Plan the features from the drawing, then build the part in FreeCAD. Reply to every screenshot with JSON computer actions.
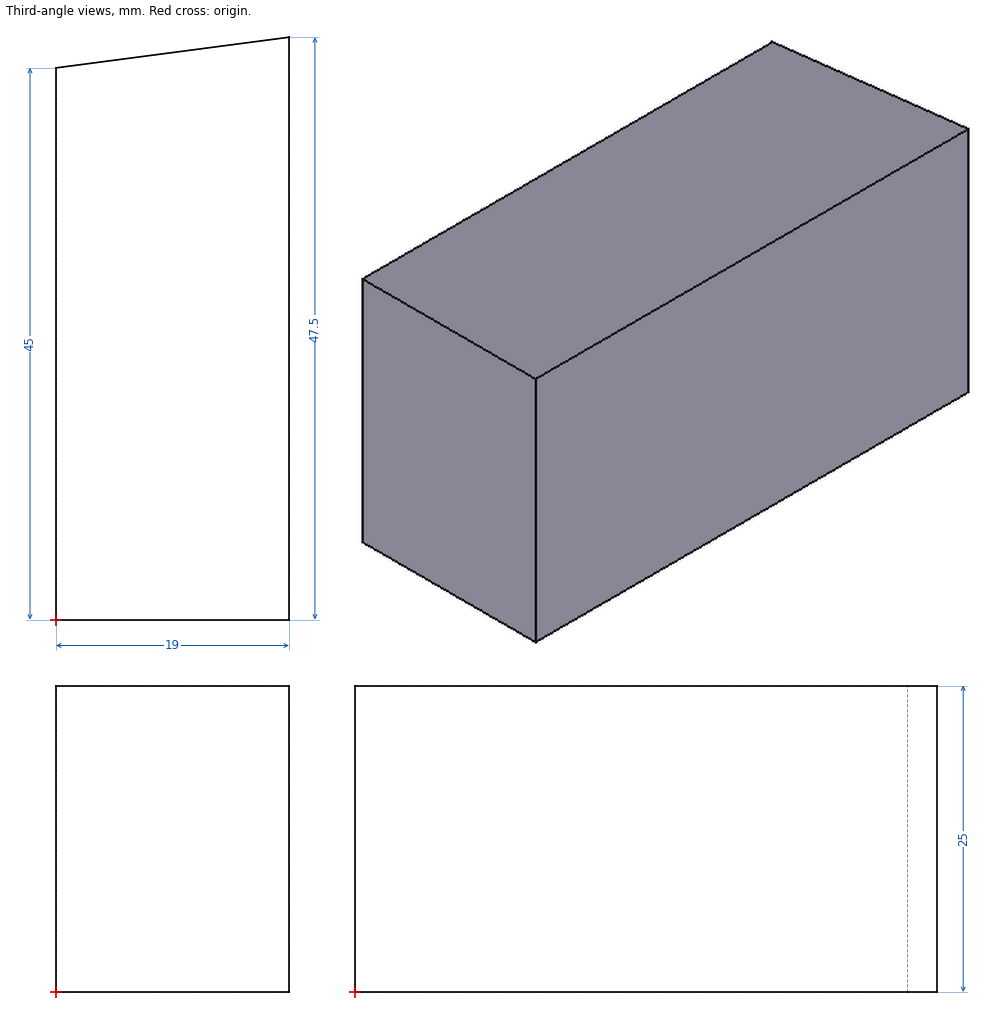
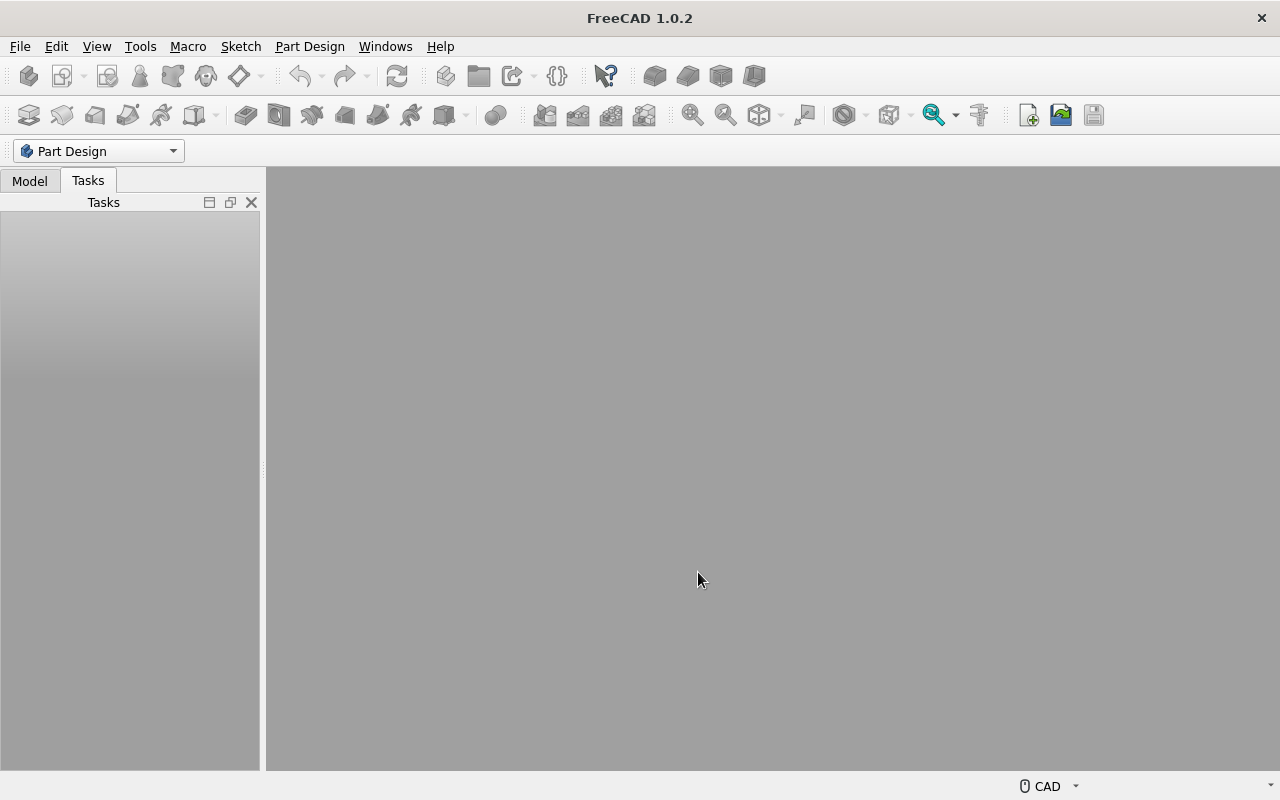
{"action": "key", "text": "ctrl+n"}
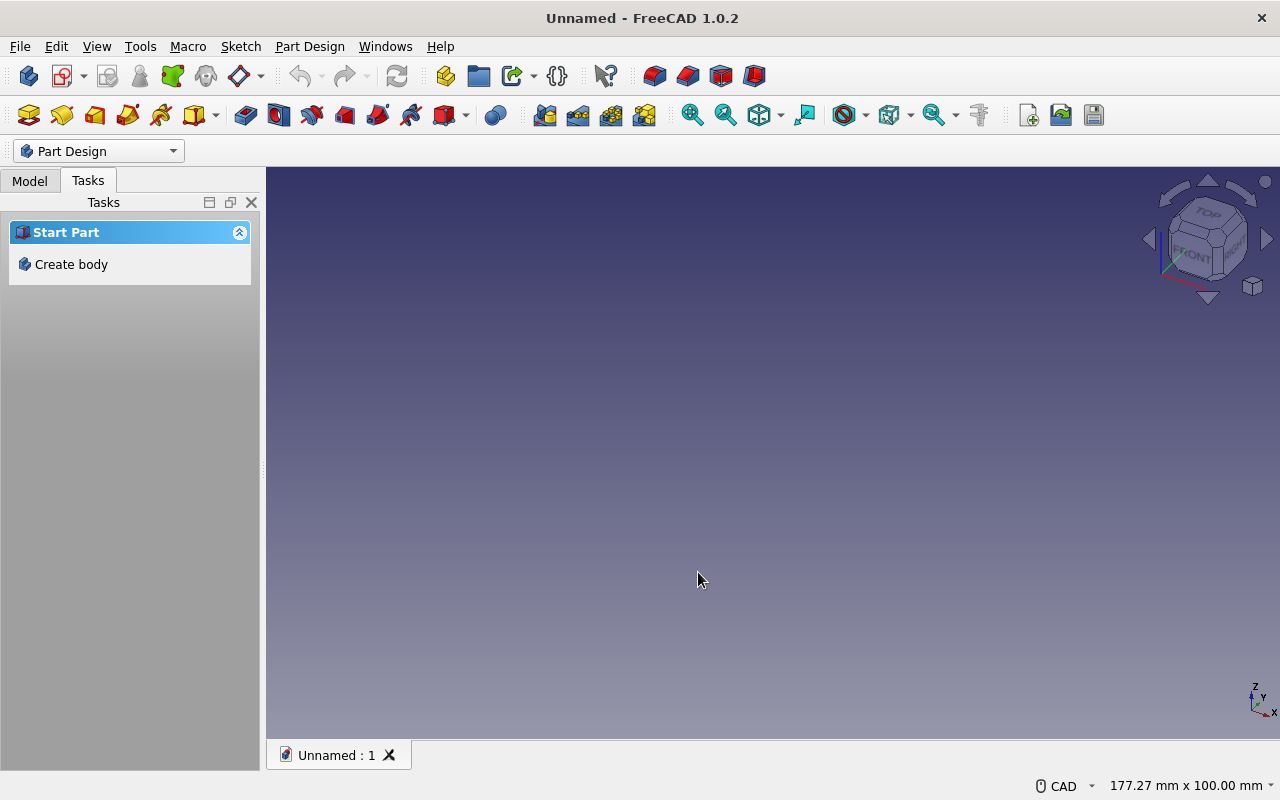
{"action": "left_click", "coordinate": [62, 76]}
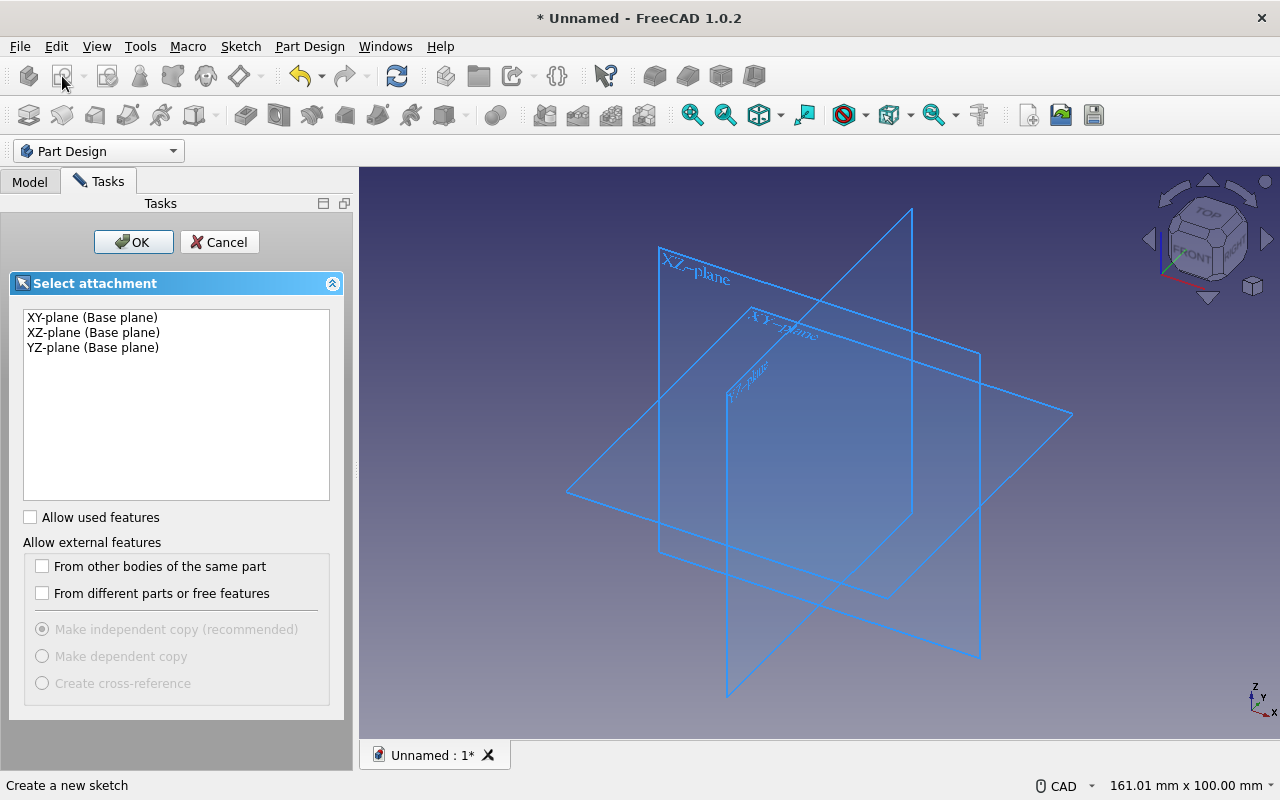
{"action": "left_click", "coordinate": [84, 318]}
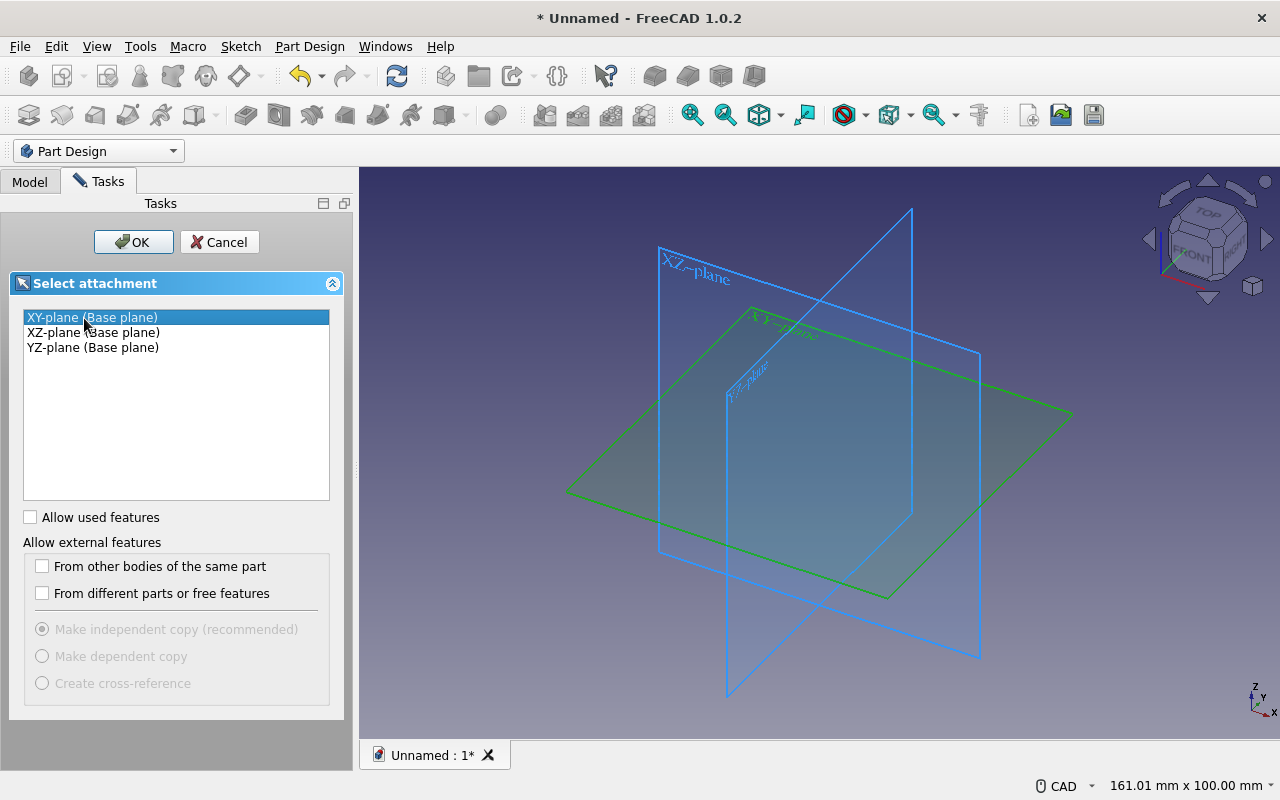
{"action": "left_click", "coordinate": [134, 242]}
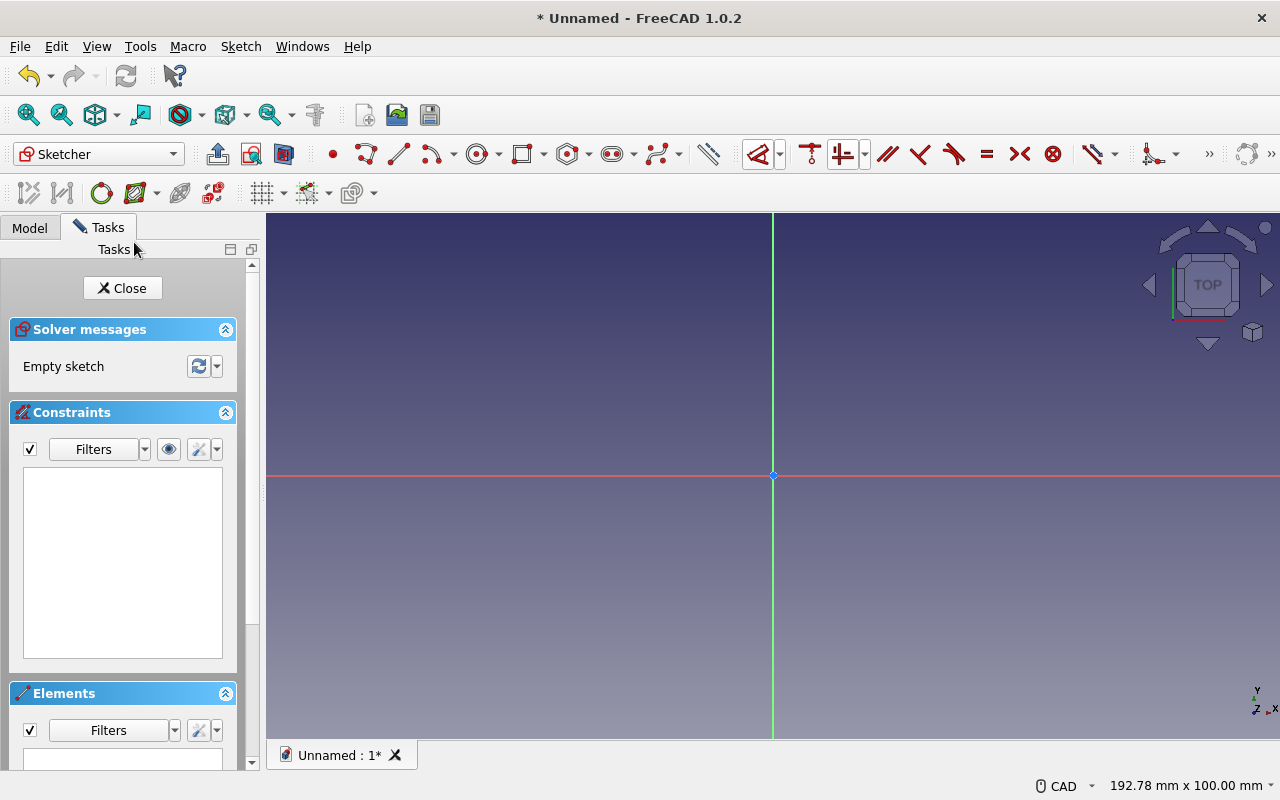
{"action": "scroll", "coordinate": [294, 711], "scroll_direction": "down", "scroll_amount": 1}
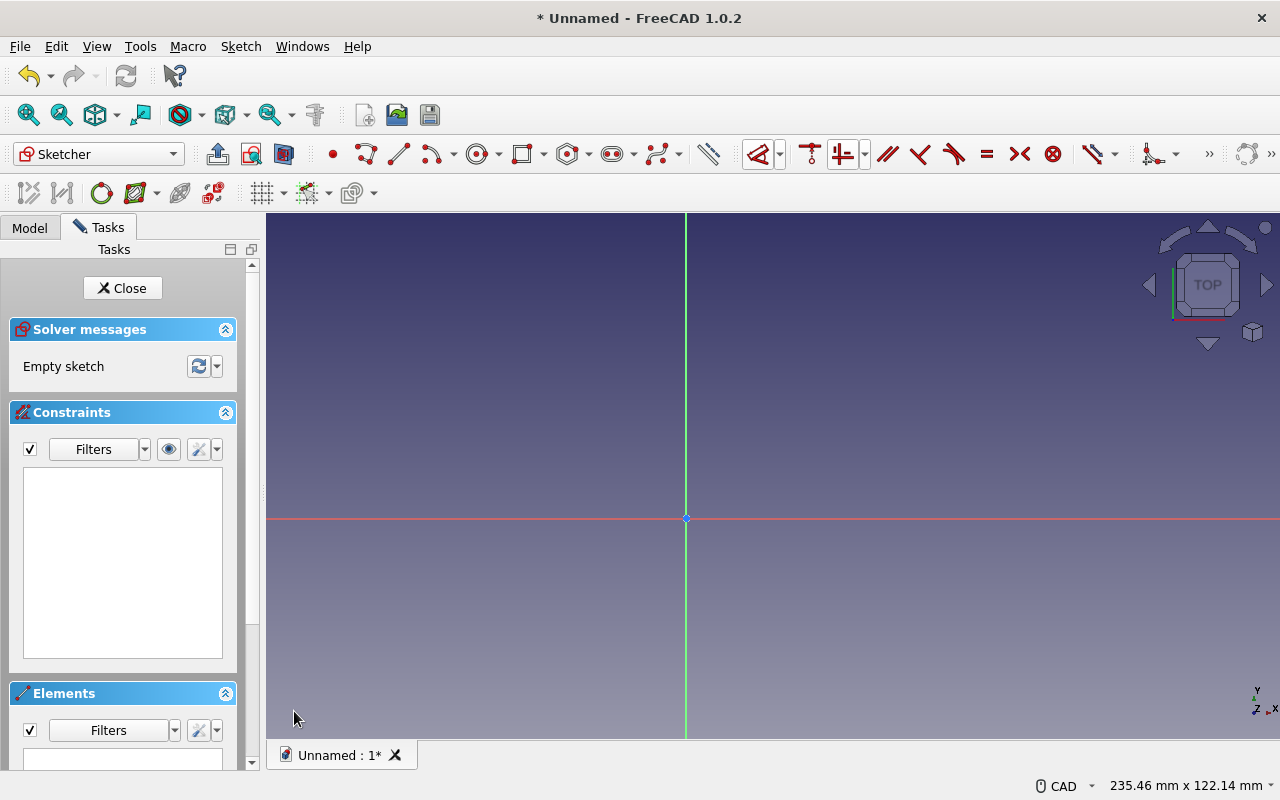
{"action": "scroll", "coordinate": [773, 295], "scroll_direction": "up", "scroll_amount": 2}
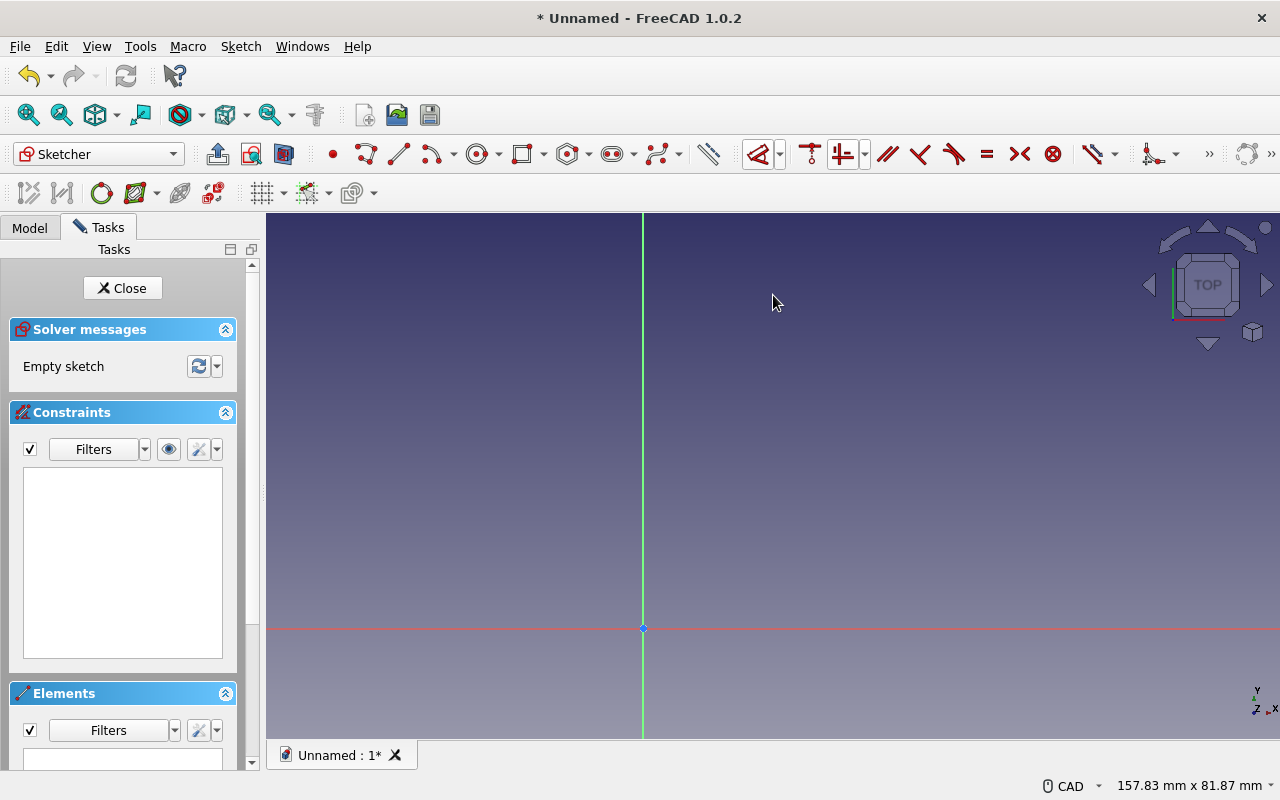
{"action": "key", "text": "g m"}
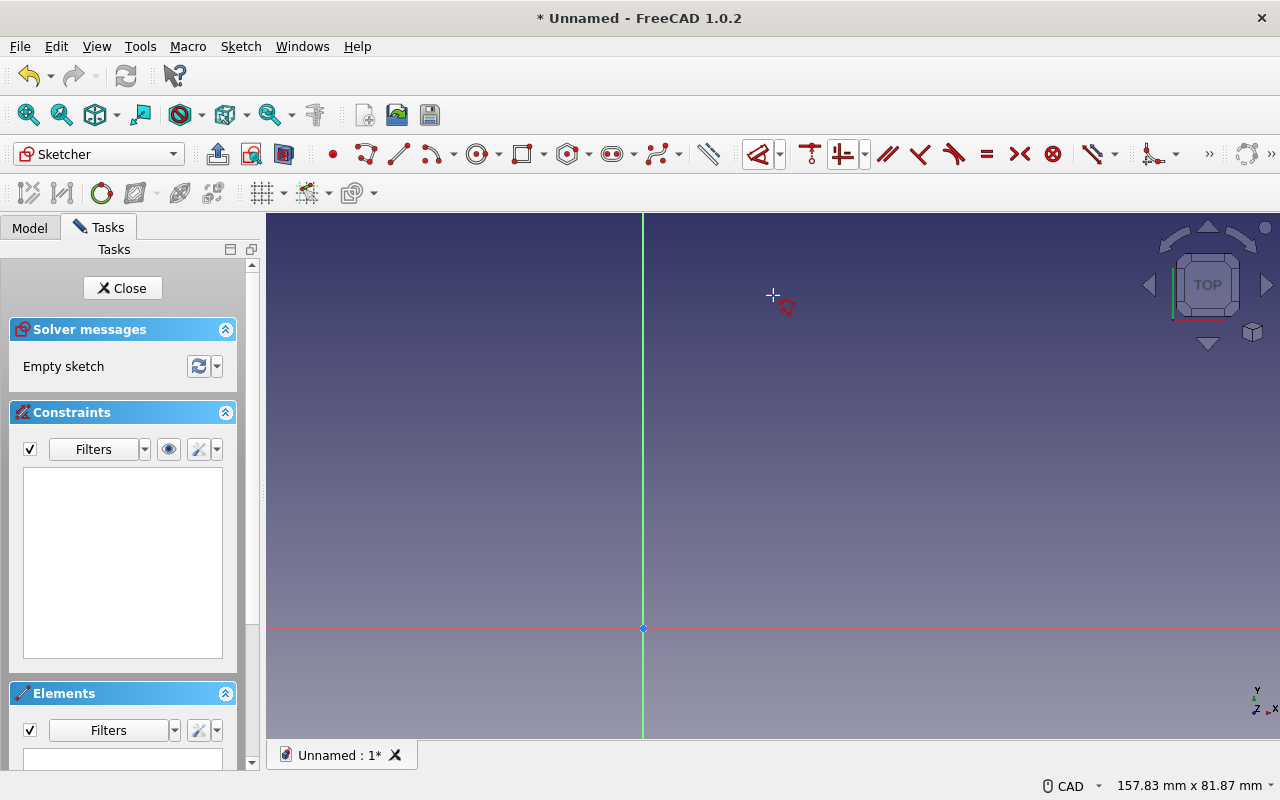
{"action": "left_click", "coordinate": [643, 629]}
{"action": "left_click", "coordinate": [765, 620]}
{"action": "left_click", "coordinate": [765, 324]}
{"action": "left_click", "coordinate": [652, 340]}
{"action": "left_click", "coordinate": [643, 629]}
{"action": "key", "text": "Escape"}
{"action": "key", "text": "Escape"}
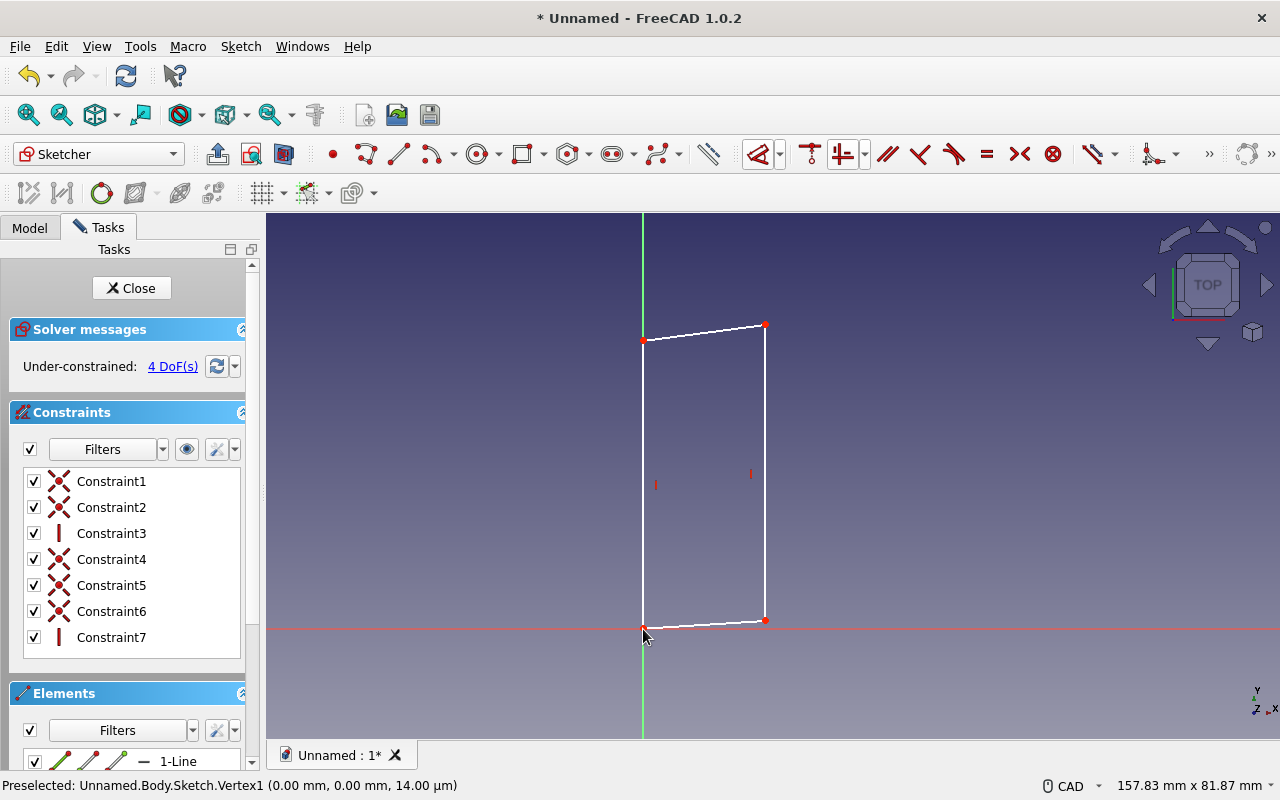
{"action": "left_click", "coordinate": [680, 626]}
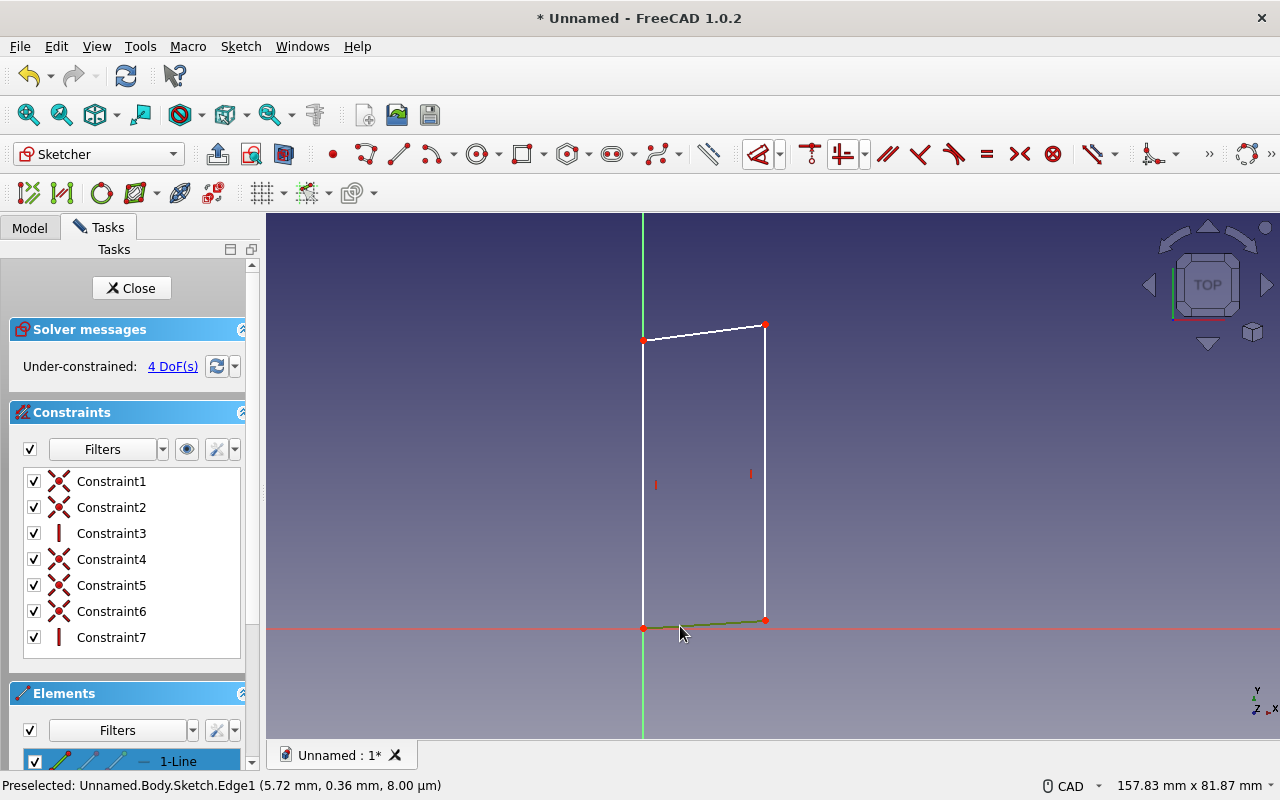
{"action": "key", "text": "h"}